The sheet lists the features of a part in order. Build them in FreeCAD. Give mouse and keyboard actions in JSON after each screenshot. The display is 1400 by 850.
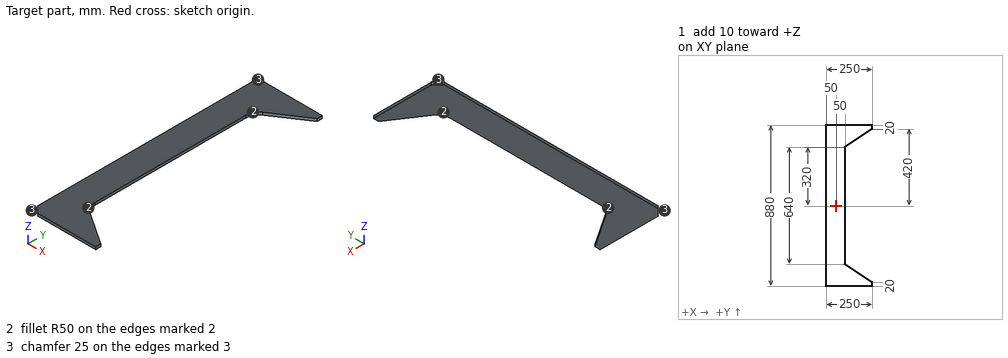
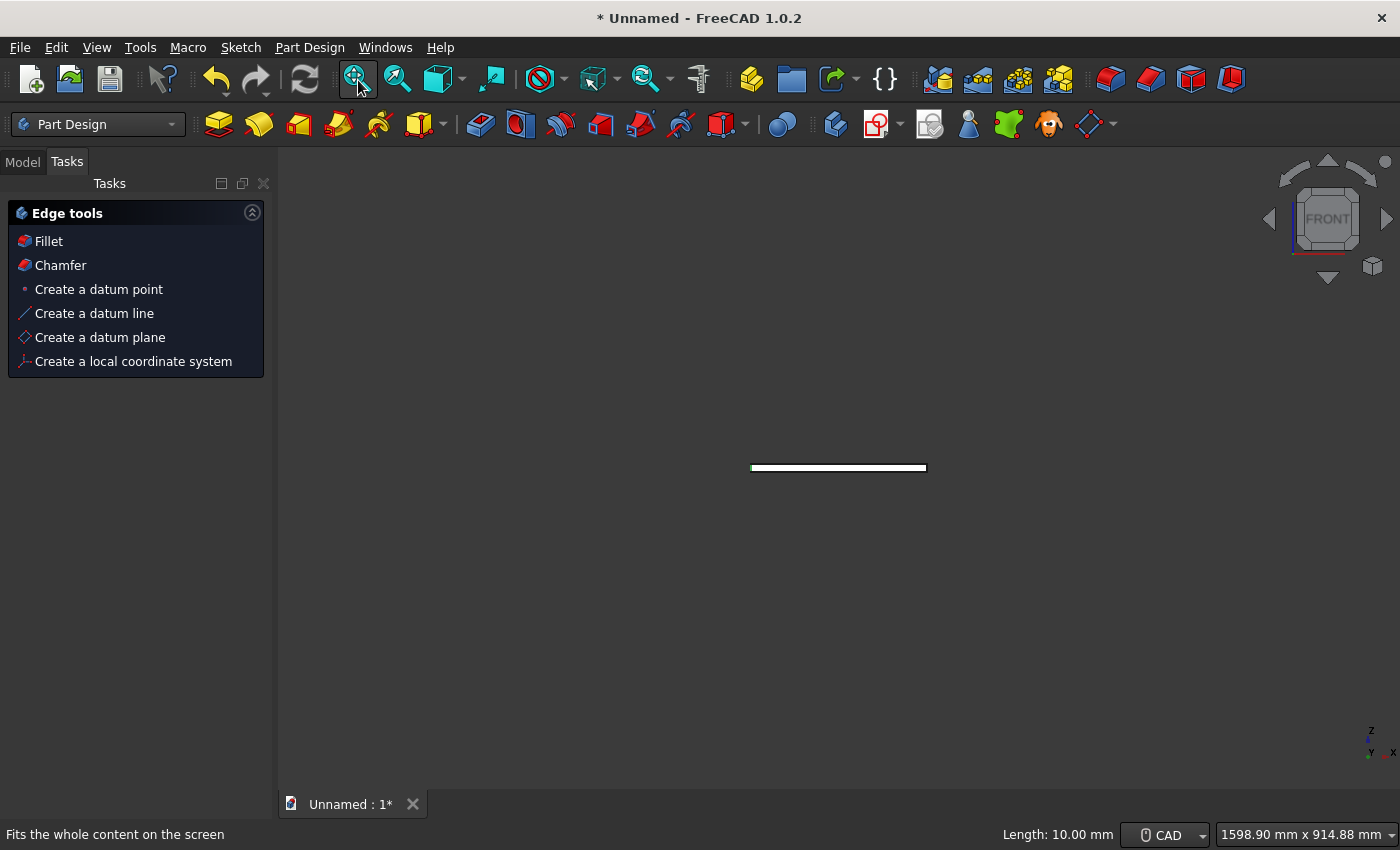
{"action": "scroll", "coordinate": [751, 467], "scroll_direction": "up", "scroll_amount": 9}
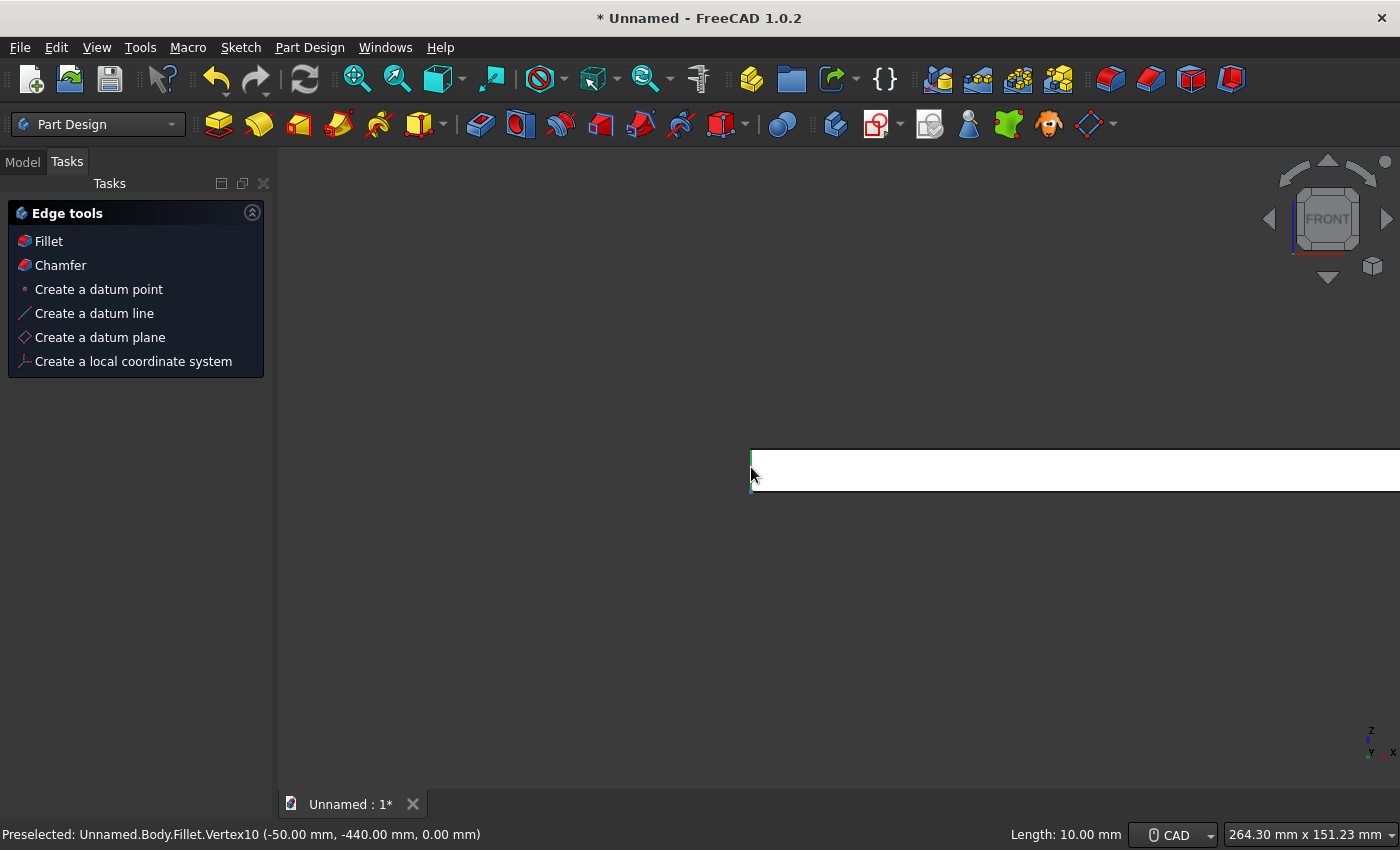
{"action": "key", "text": "v f"}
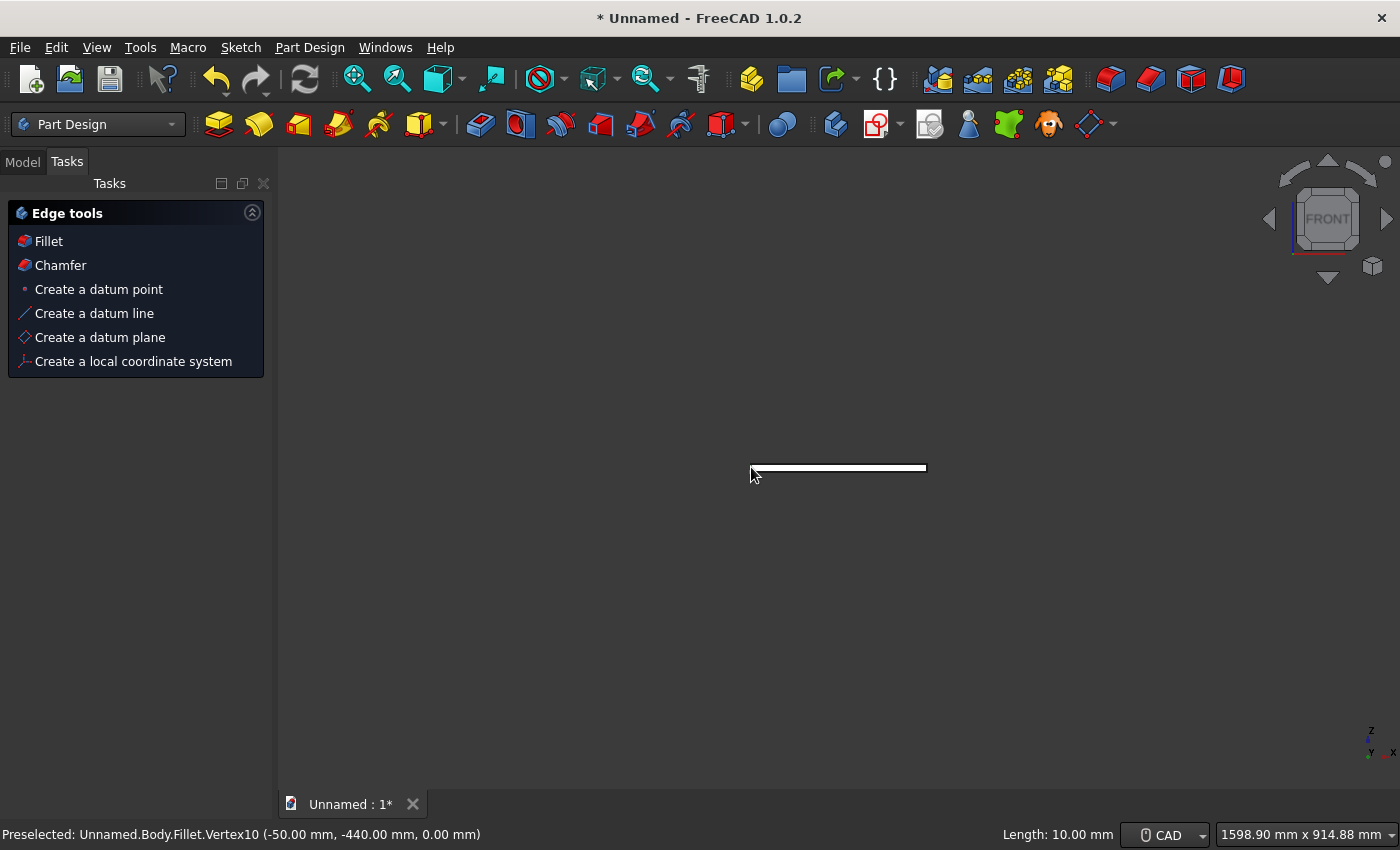
{"action": "key", "text": "3"}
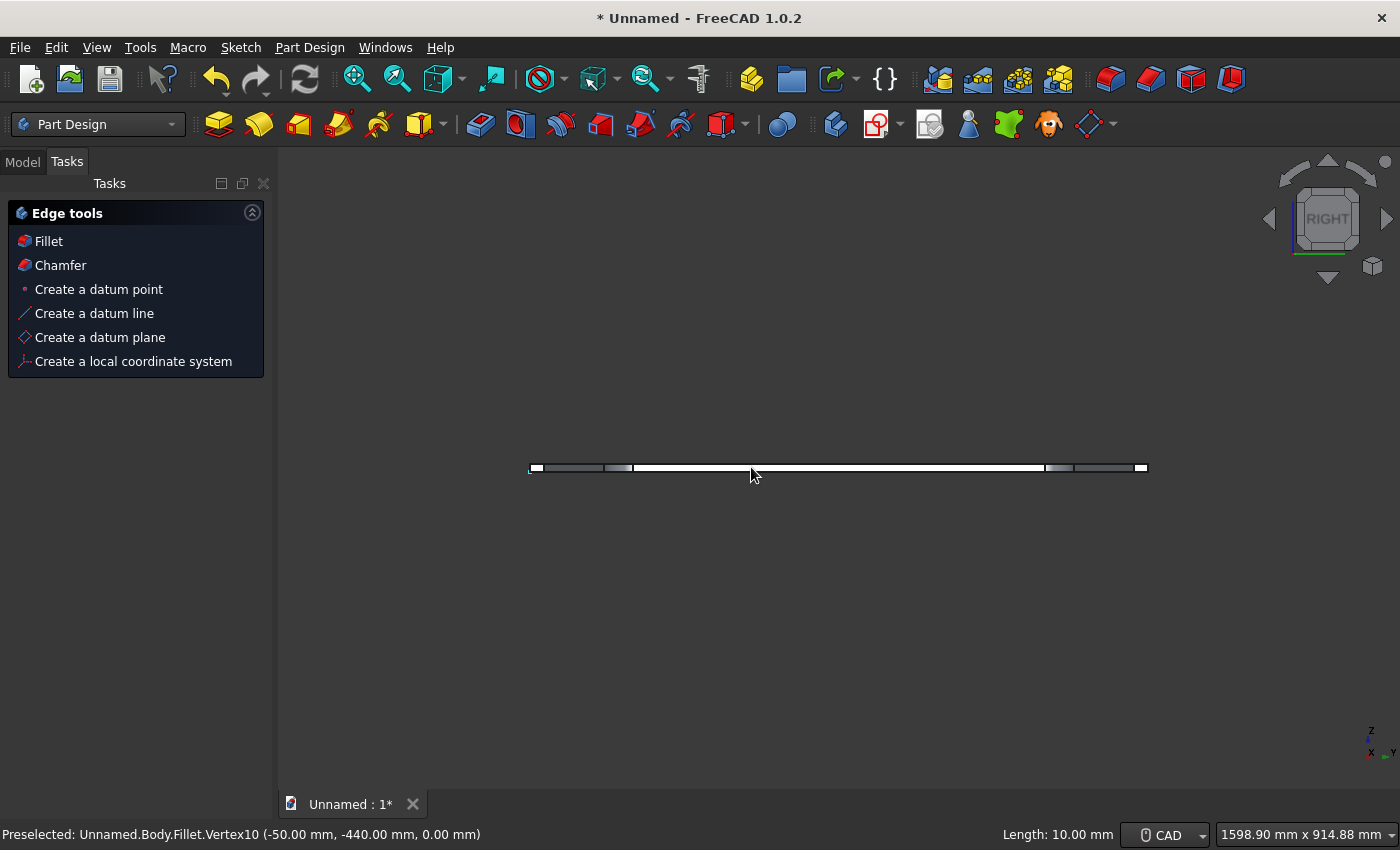
{"action": "scroll", "coordinate": [1148, 467], "scroll_direction": "up", "scroll_amount": 9}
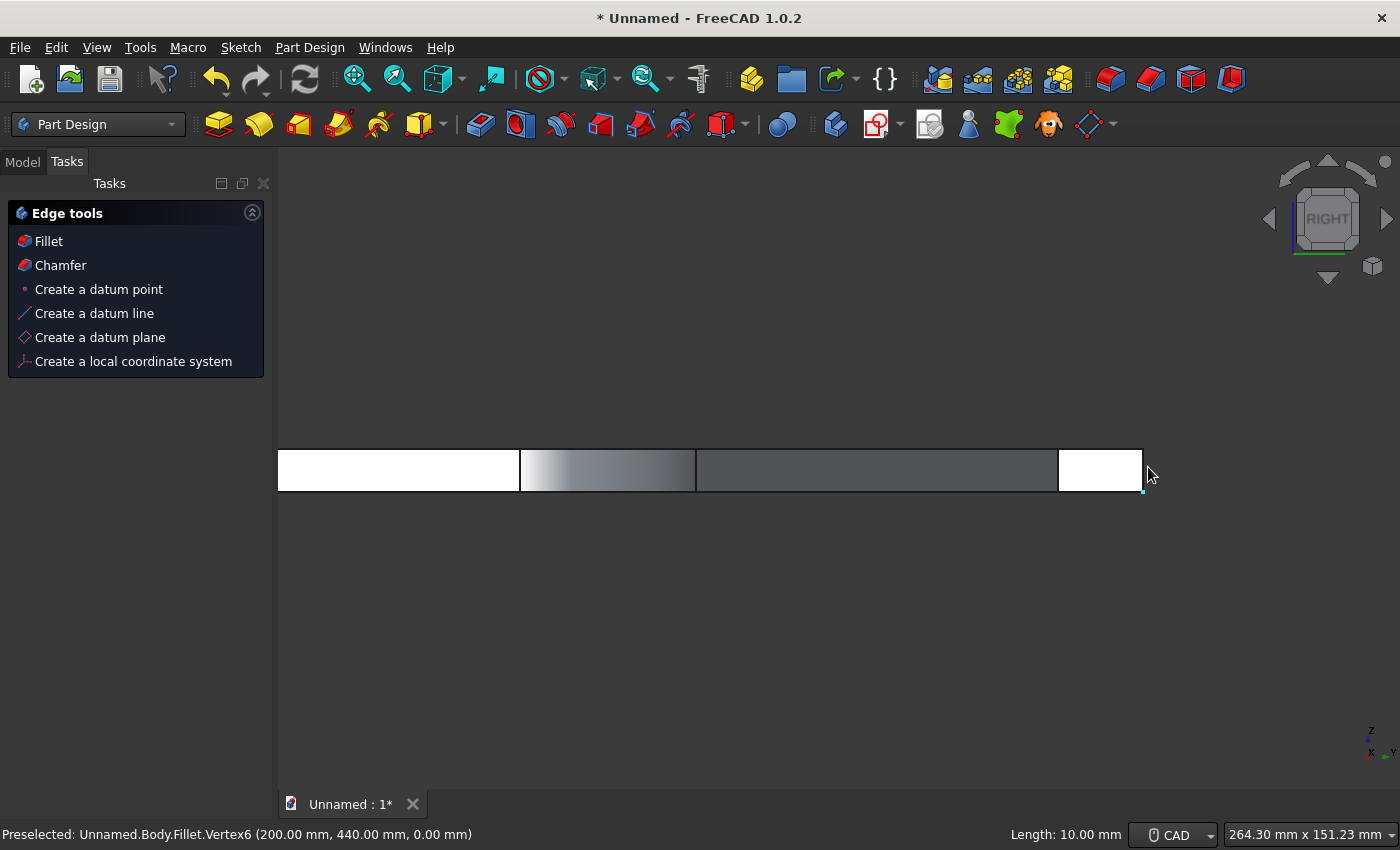
{"action": "key", "text": "v f"}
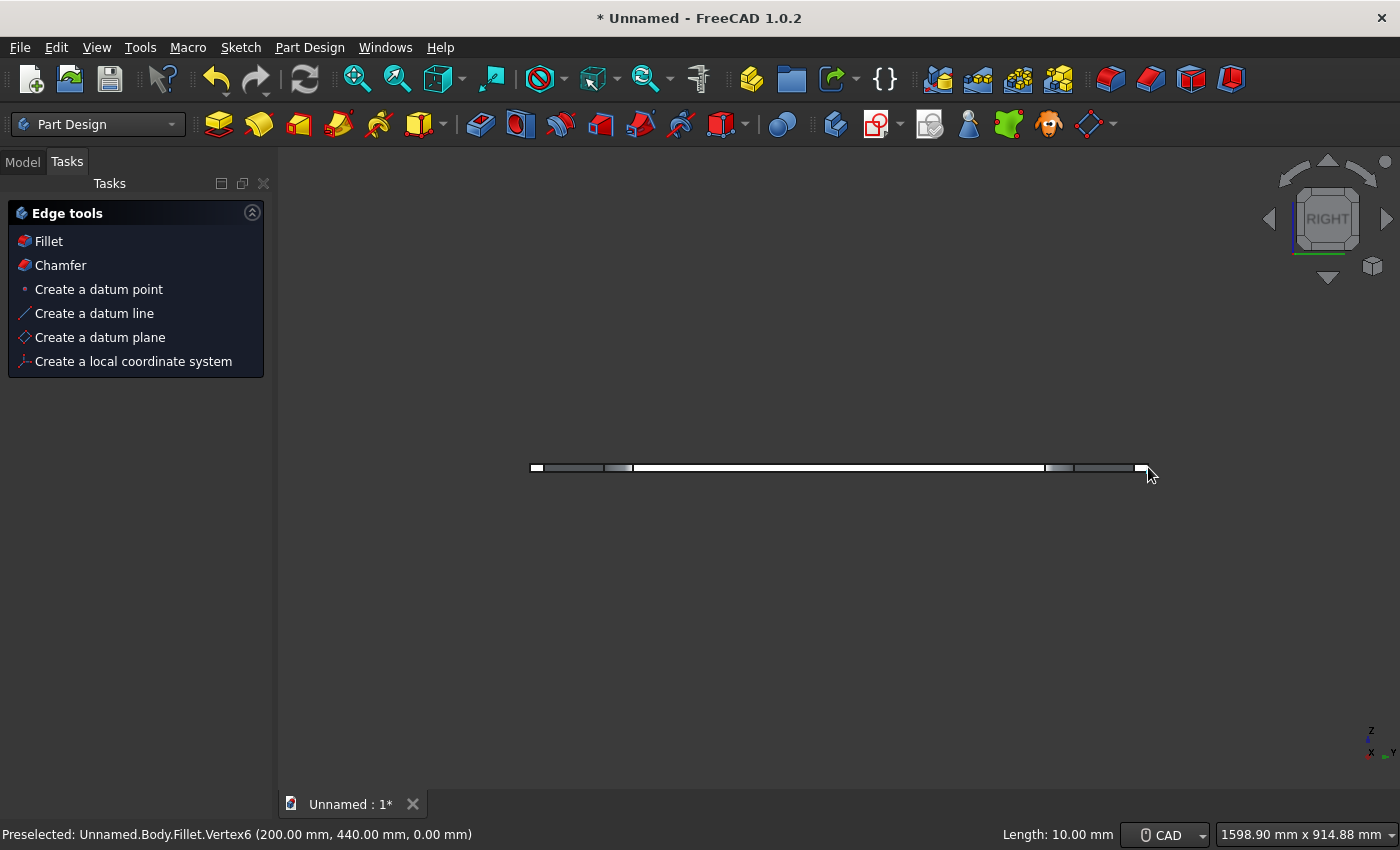
{"action": "key", "text": "5"}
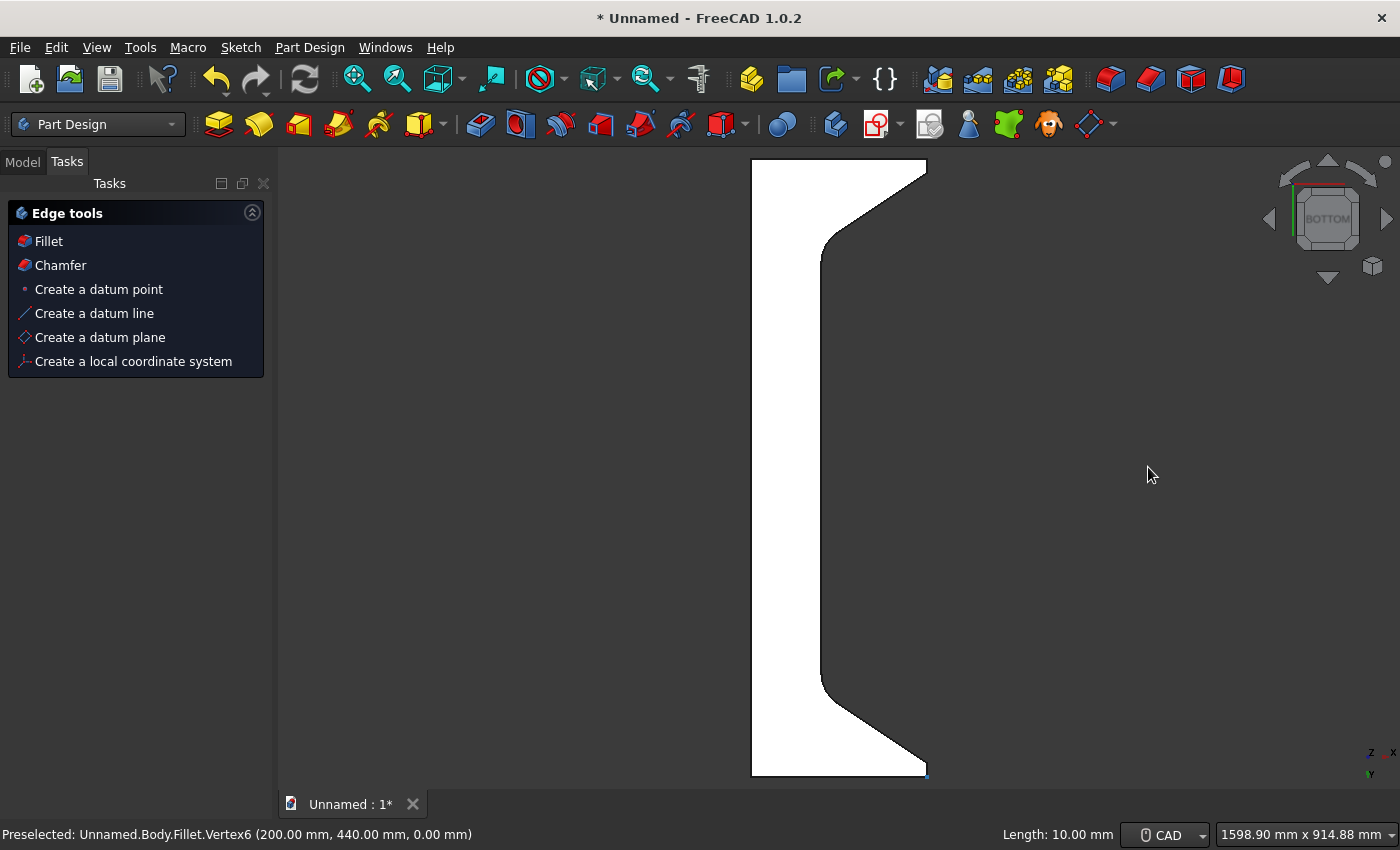
{"action": "key", "text": "4"}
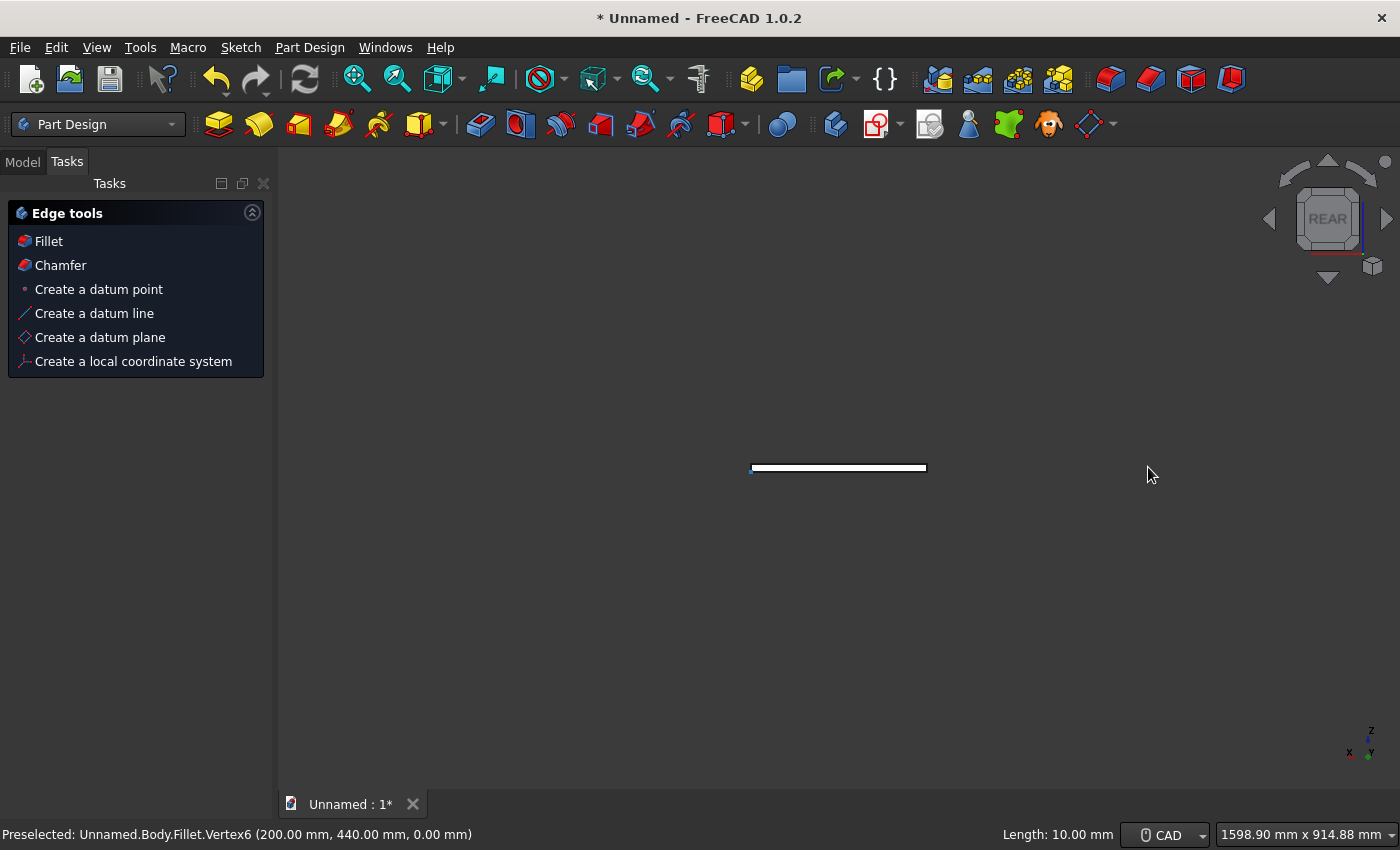
{"action": "key", "text": "v f"}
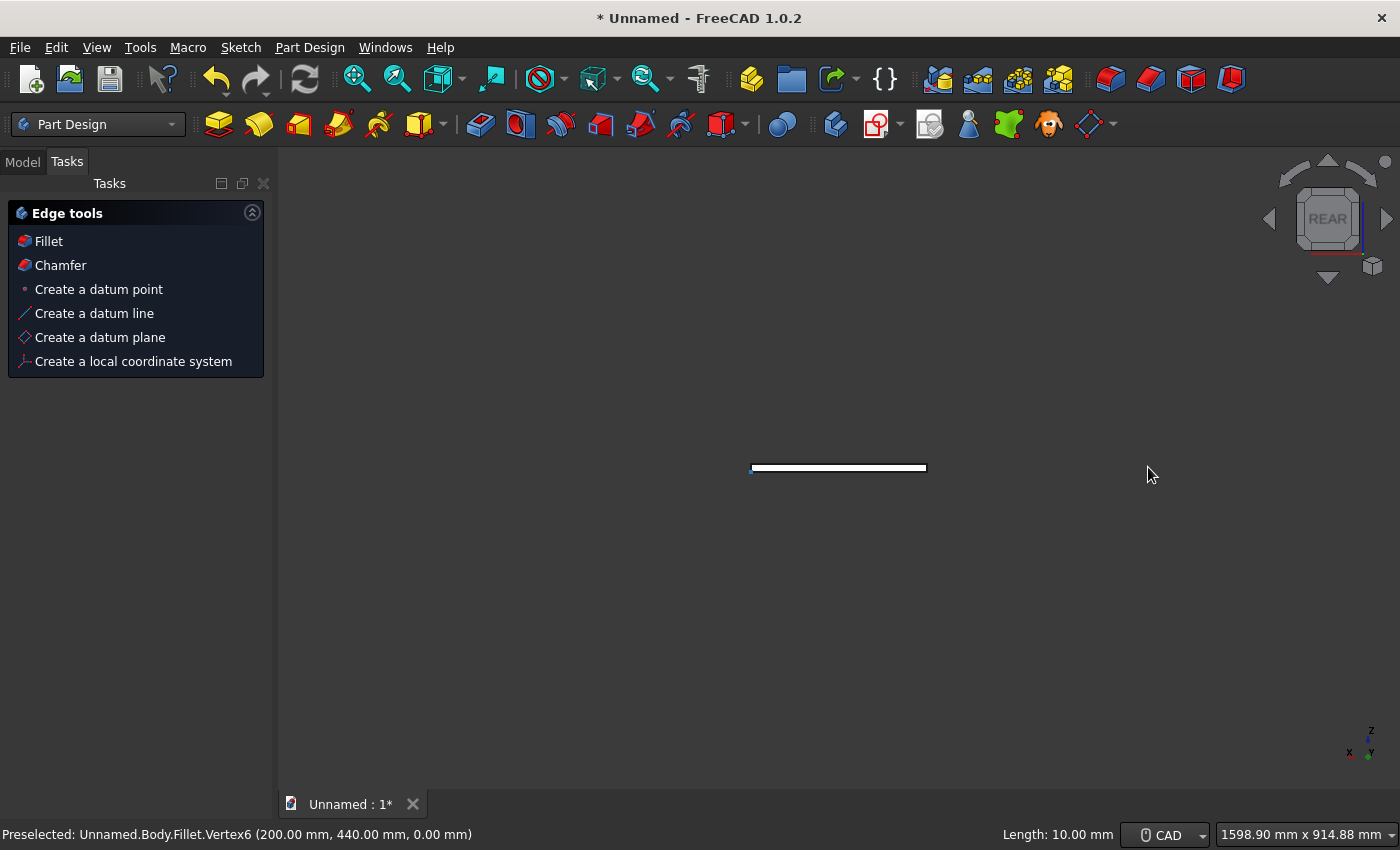
{"action": "scroll", "coordinate": [927, 467], "scroll_direction": "up", "scroll_amount": 9}